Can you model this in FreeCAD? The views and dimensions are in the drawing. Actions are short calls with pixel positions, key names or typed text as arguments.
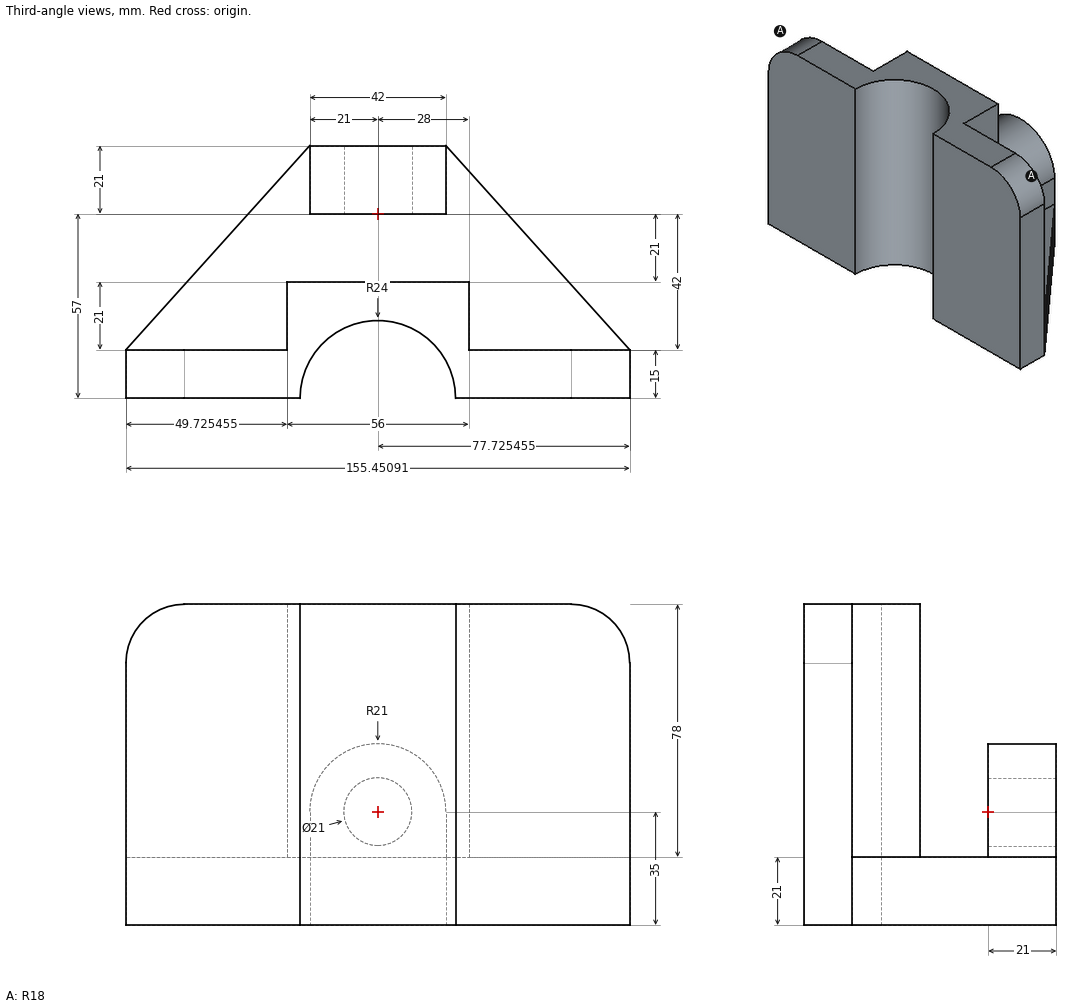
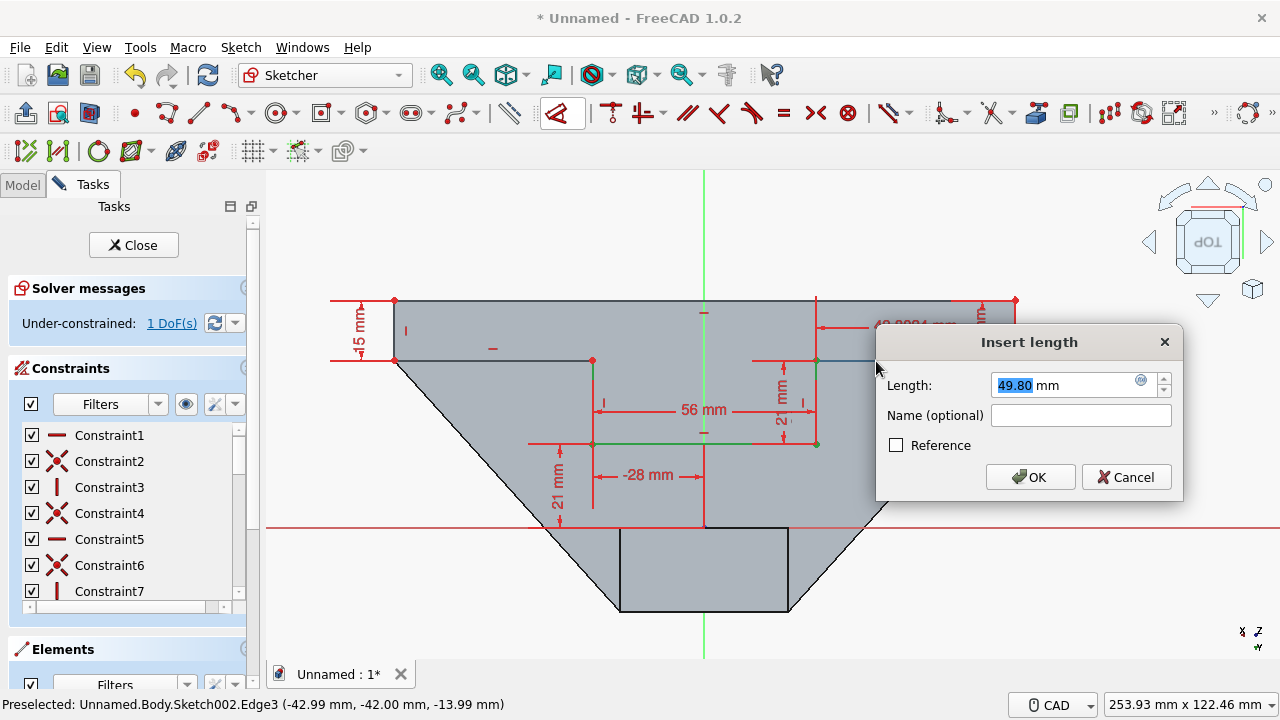
text(49.725455)
key(Return)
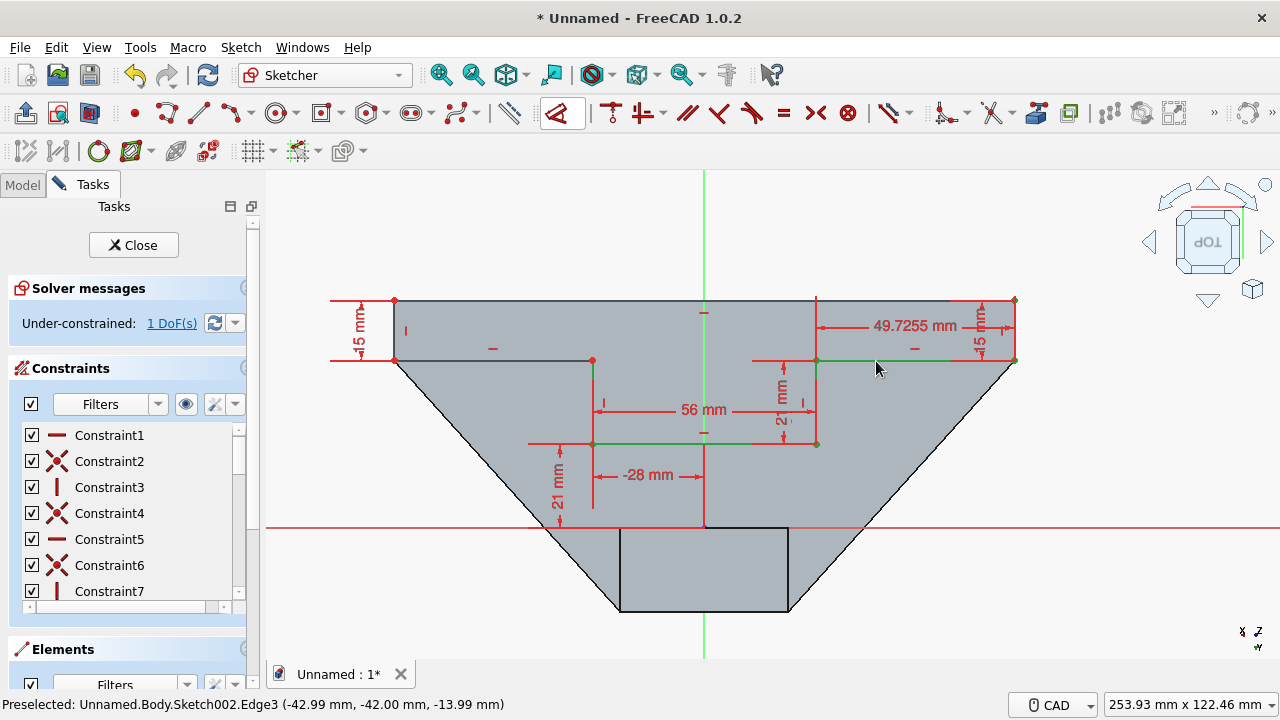
click(828, 301)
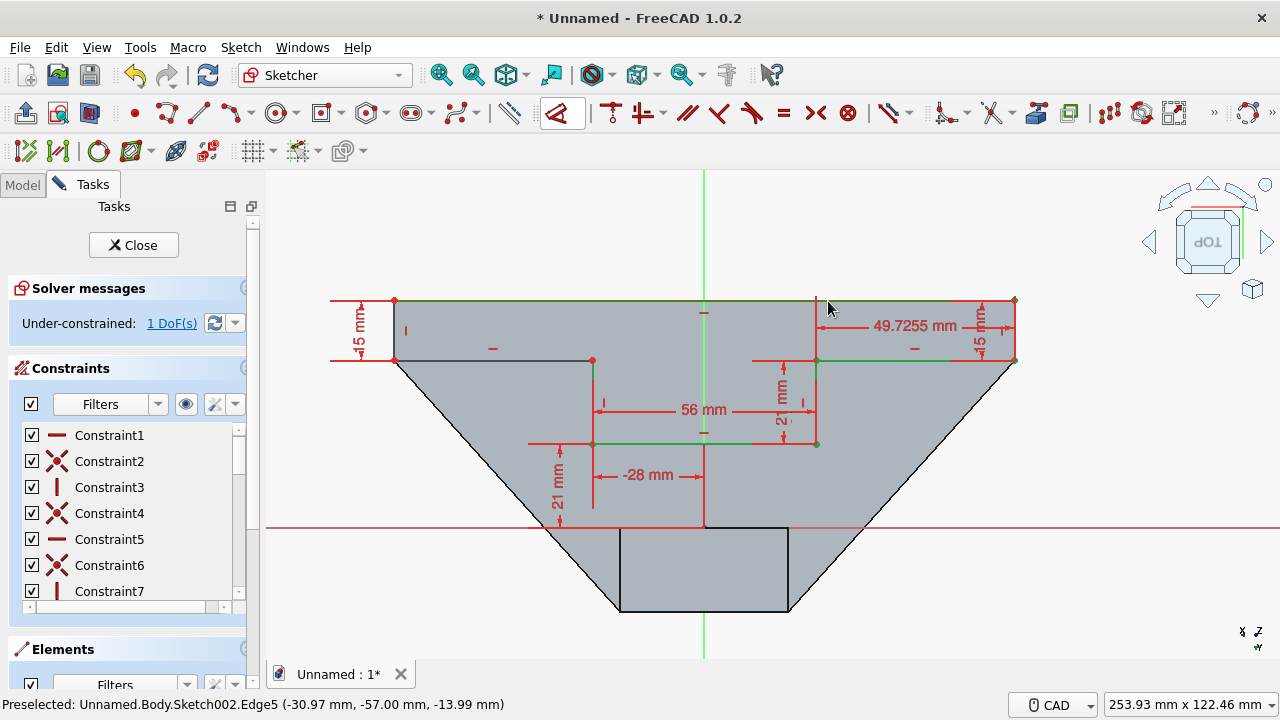
click(580, 114)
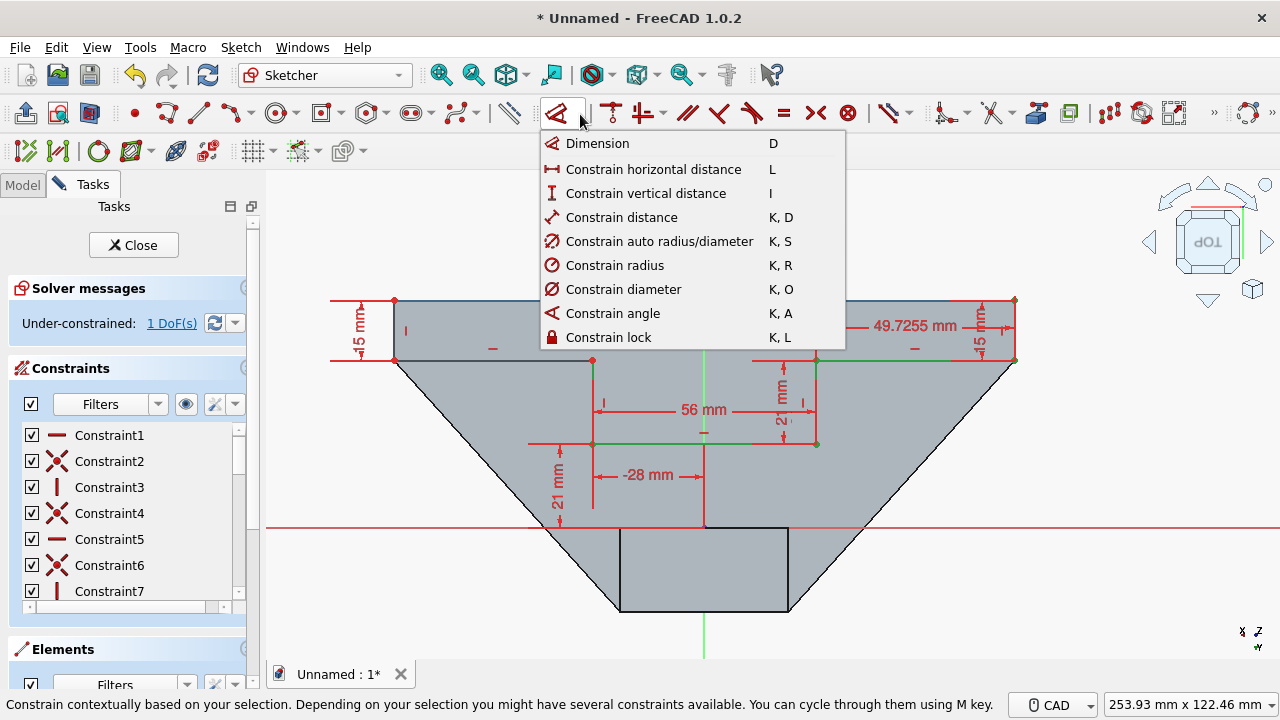
click(693, 169)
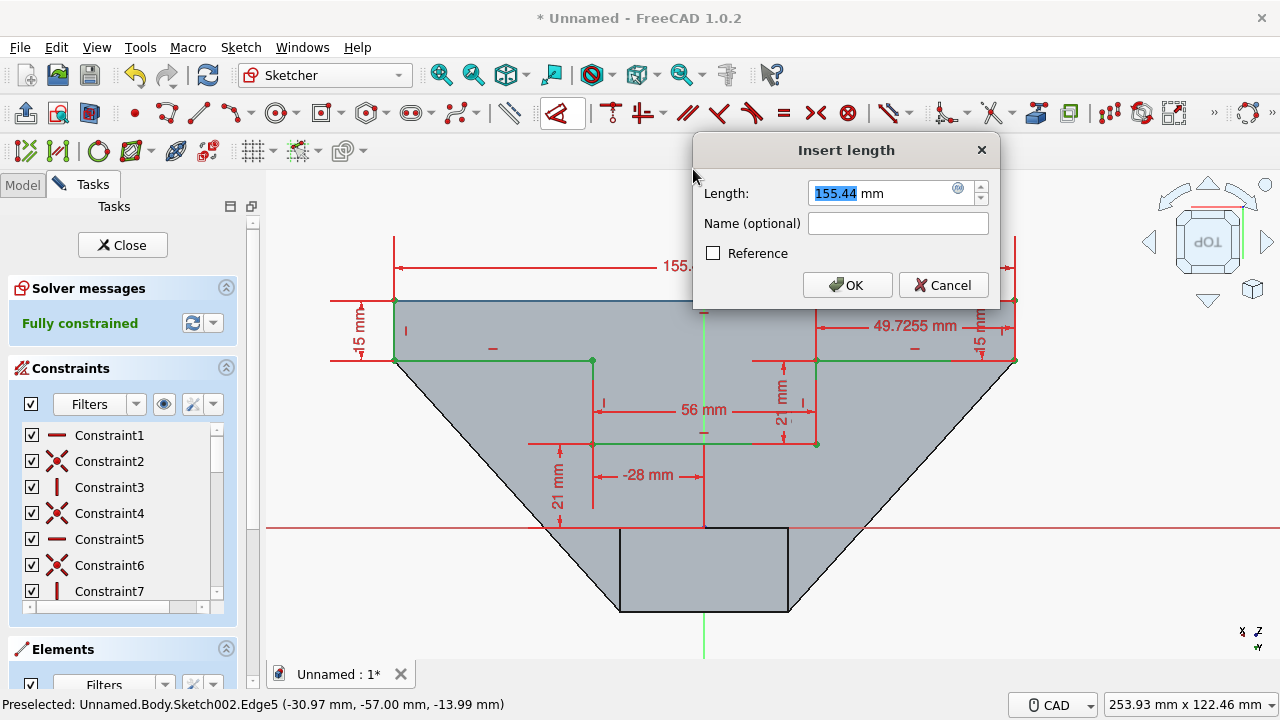
text(155.45091)
key(Return)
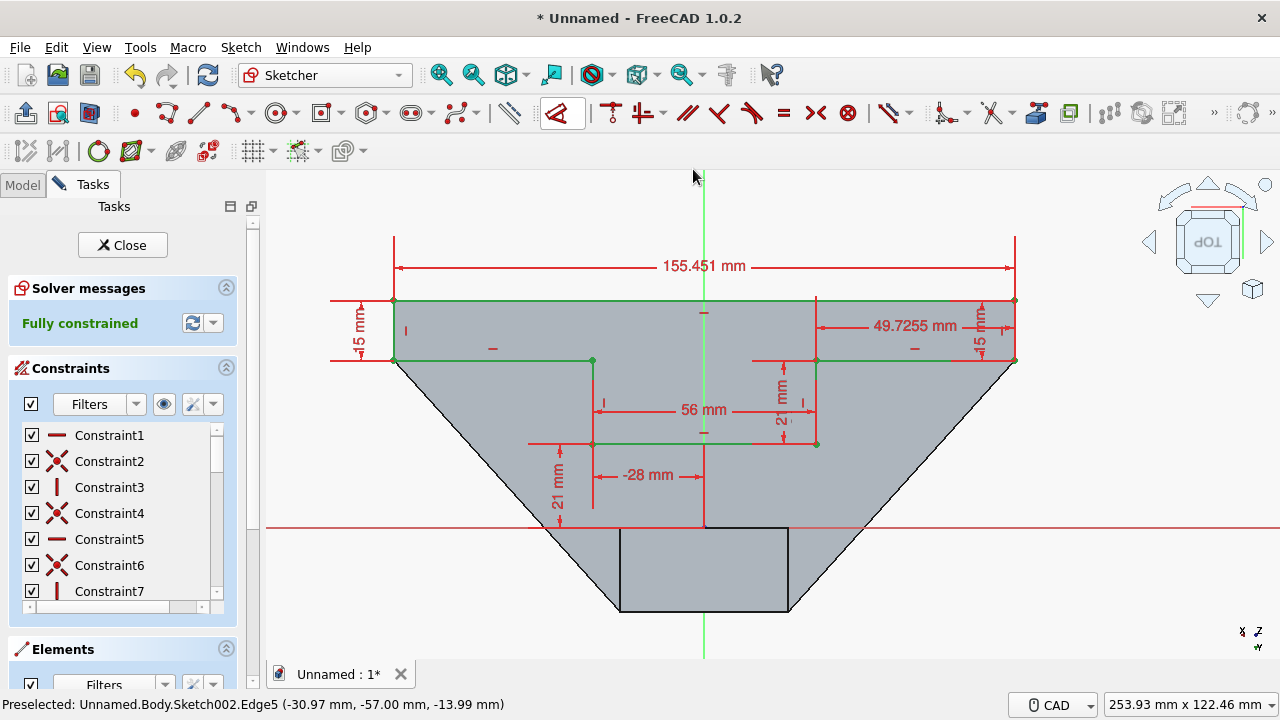
click(123, 245)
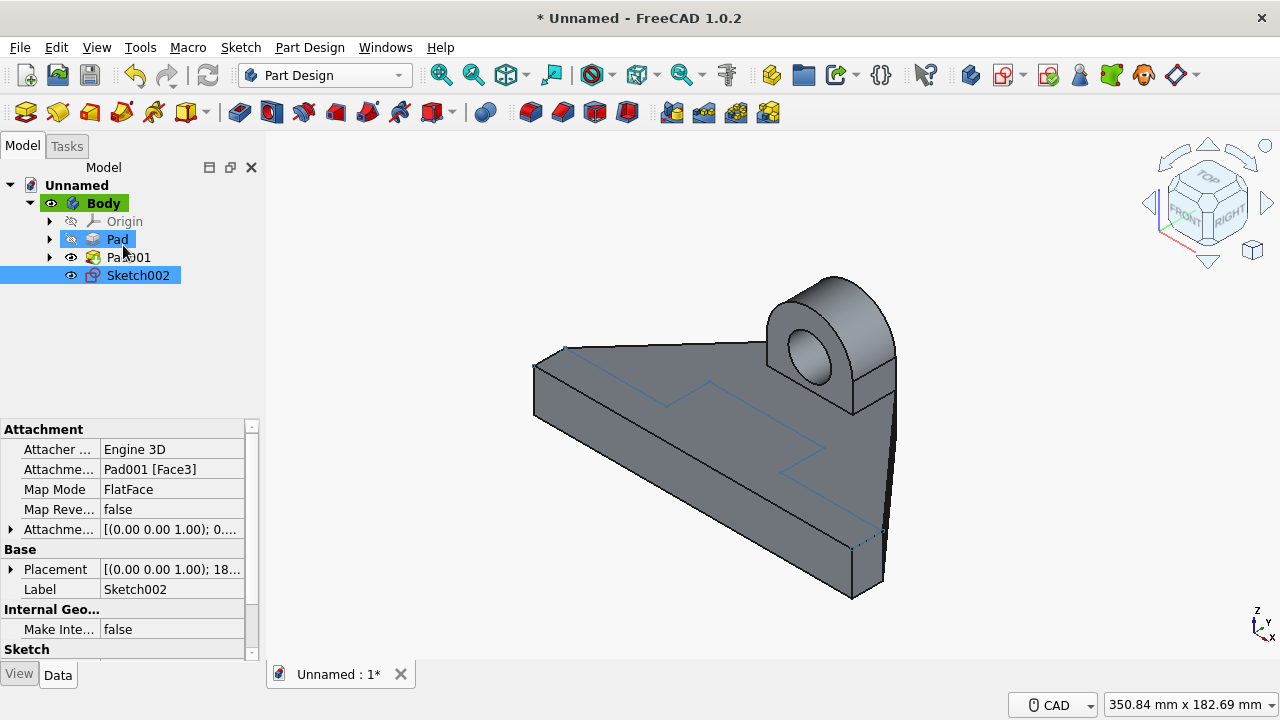
click(26, 112)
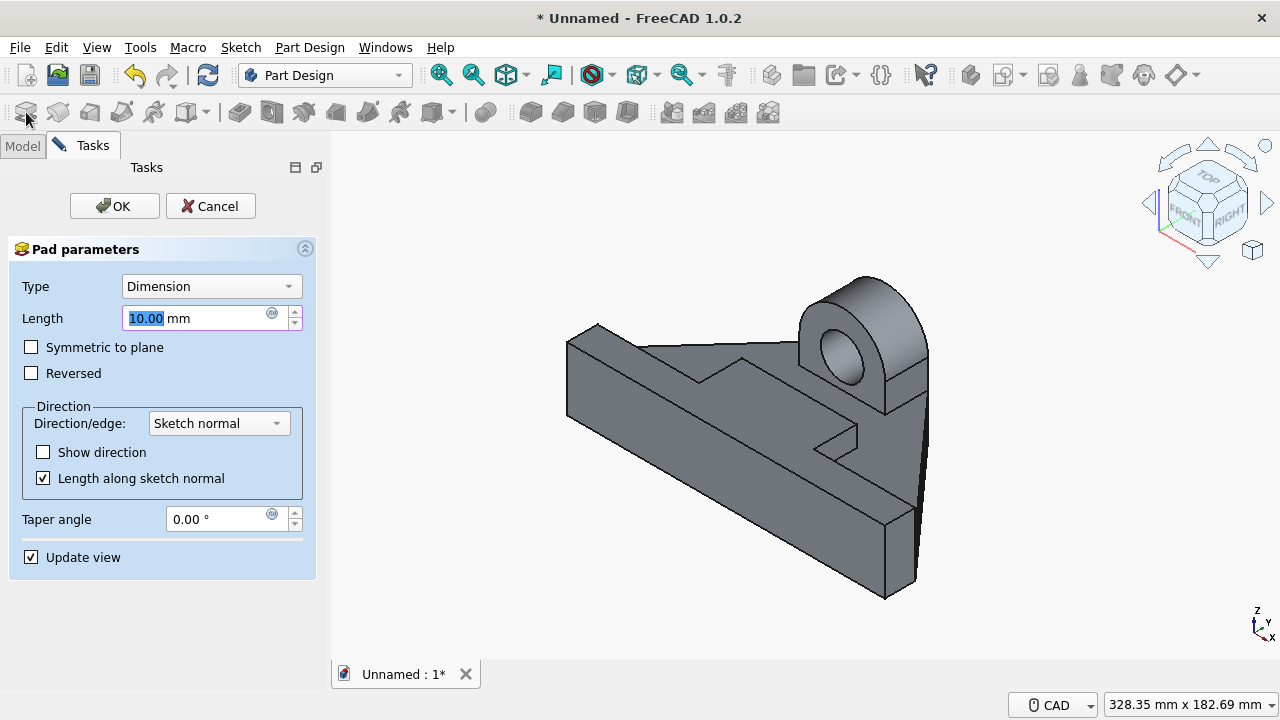
text(78)
key(Tab)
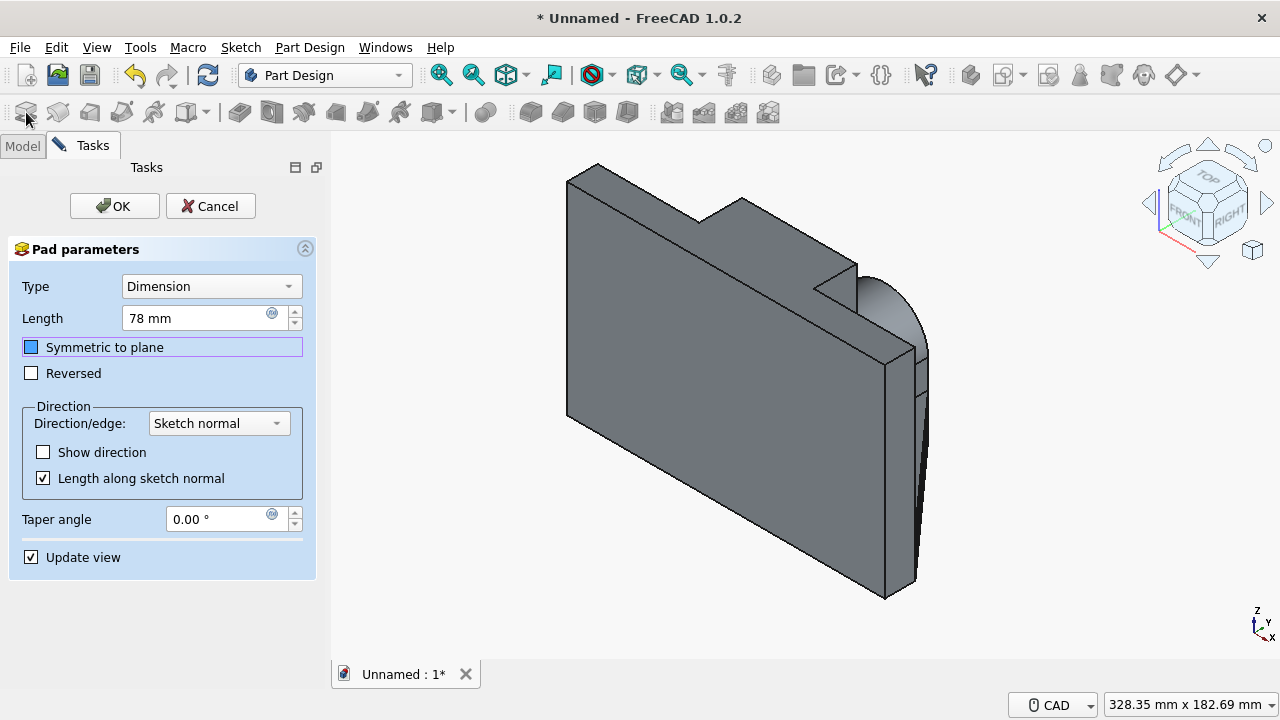
click(115, 206)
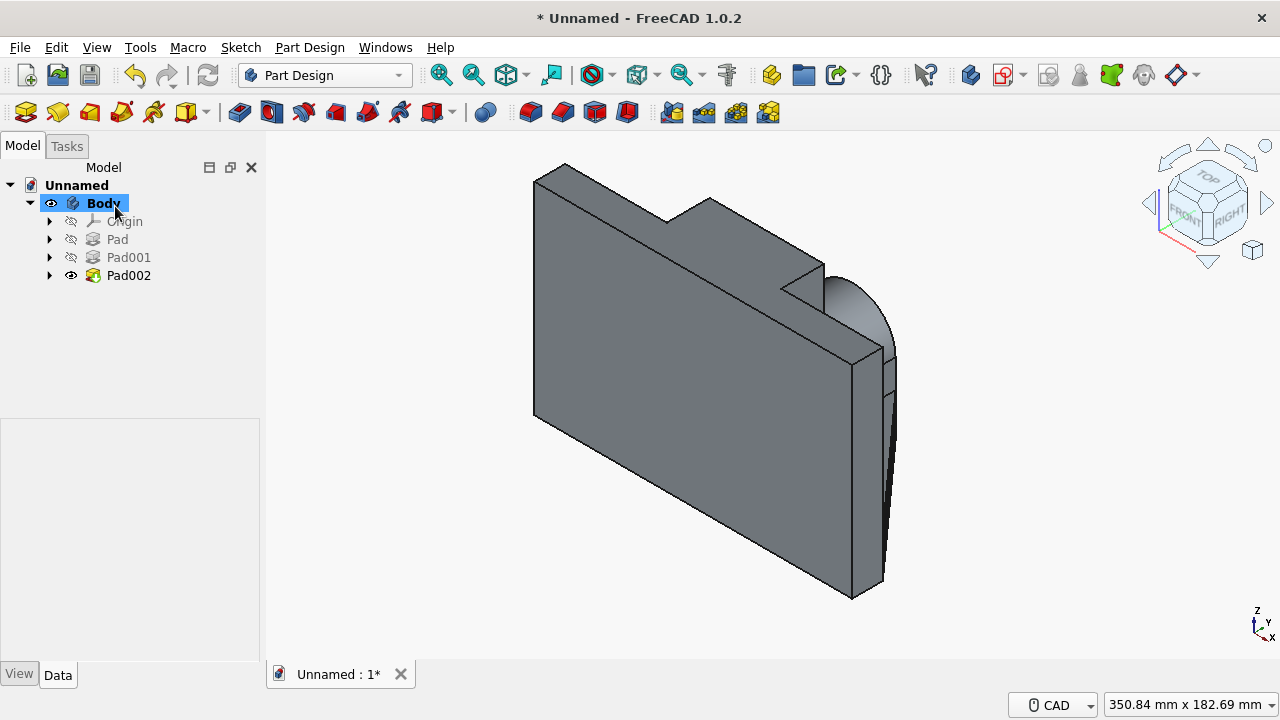
click(442, 76)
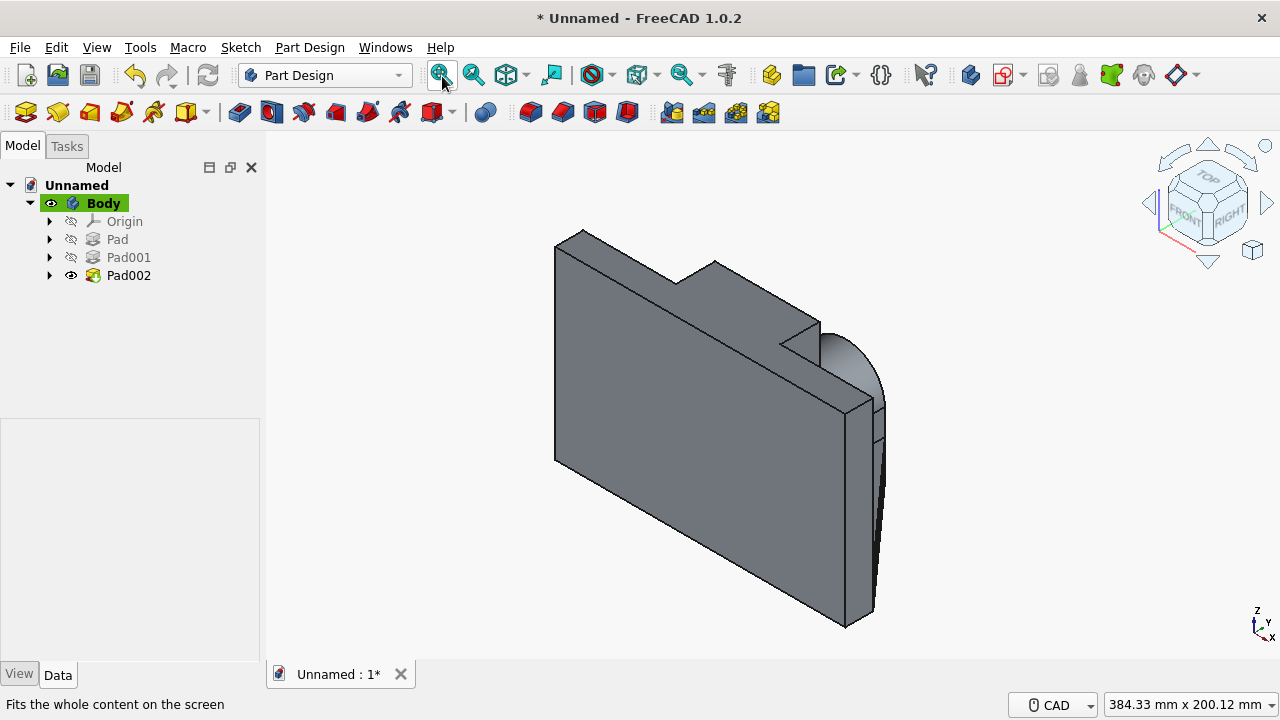
click(859, 405)